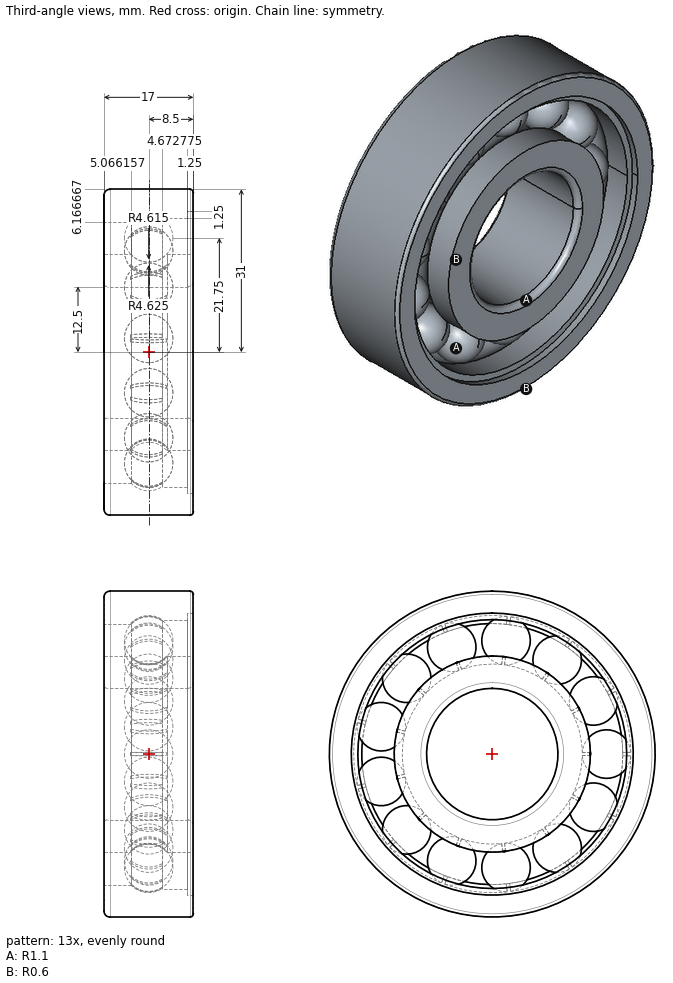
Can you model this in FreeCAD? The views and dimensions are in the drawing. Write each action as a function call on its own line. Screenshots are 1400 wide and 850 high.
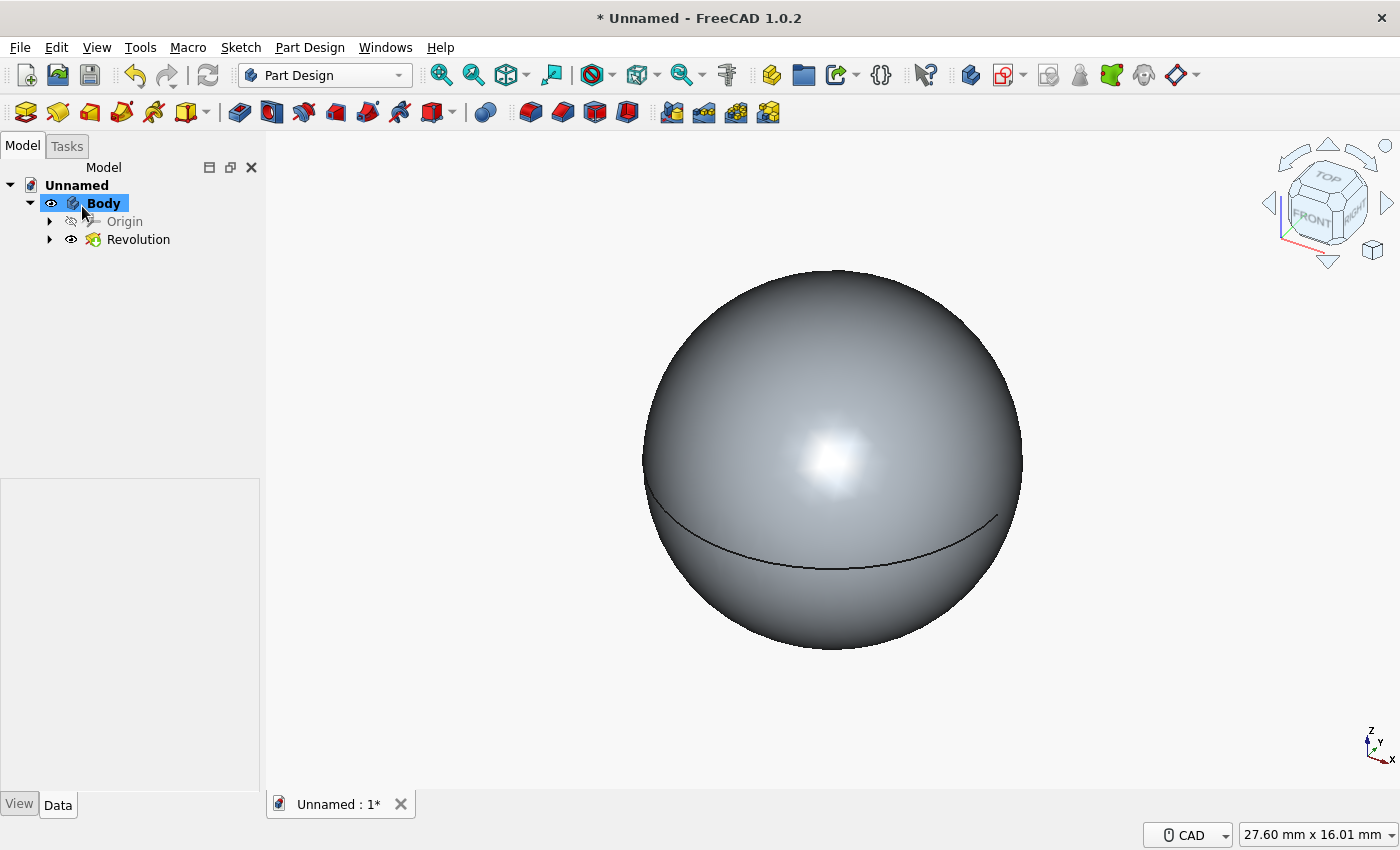
click(1004, 76)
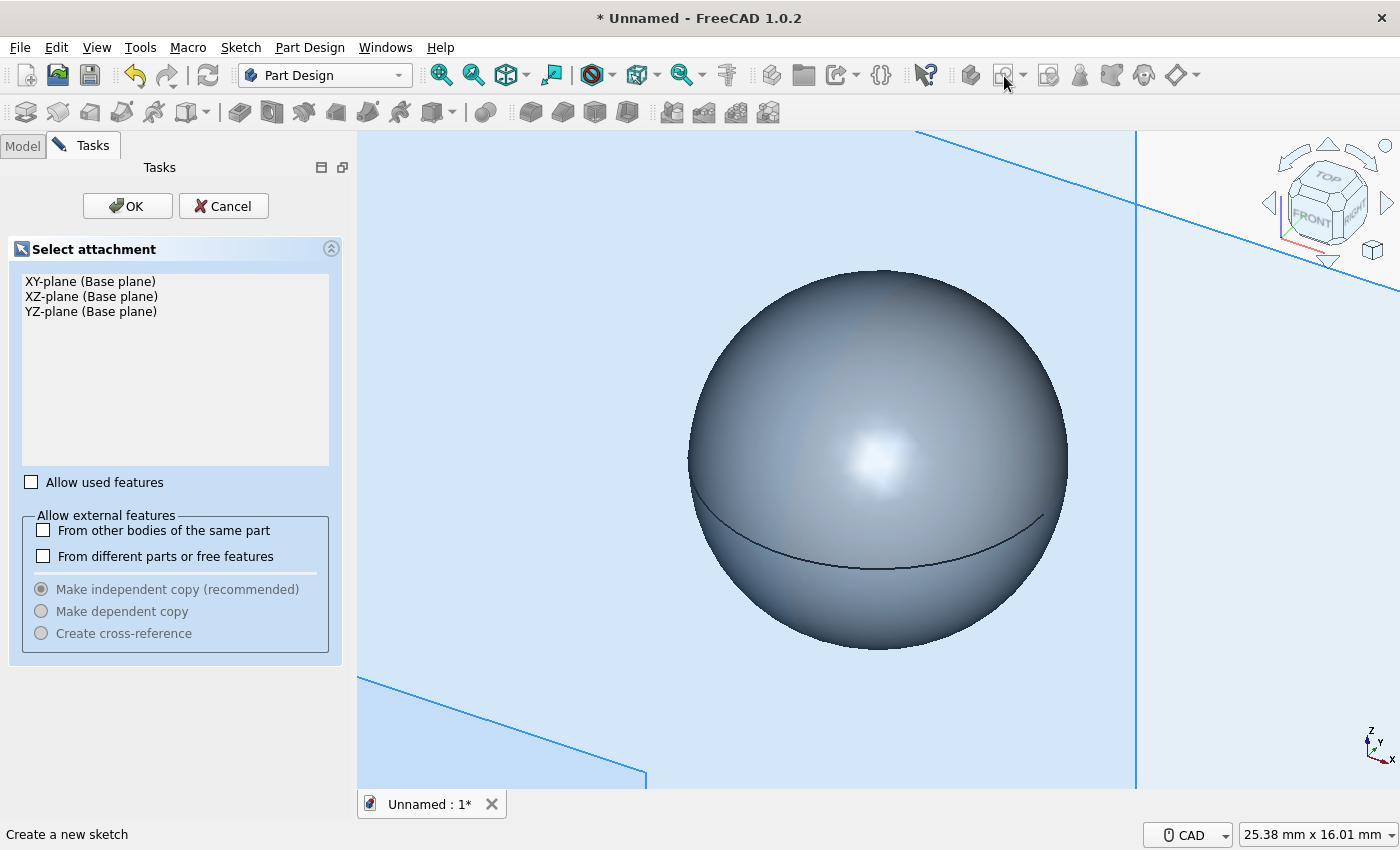
click(82, 282)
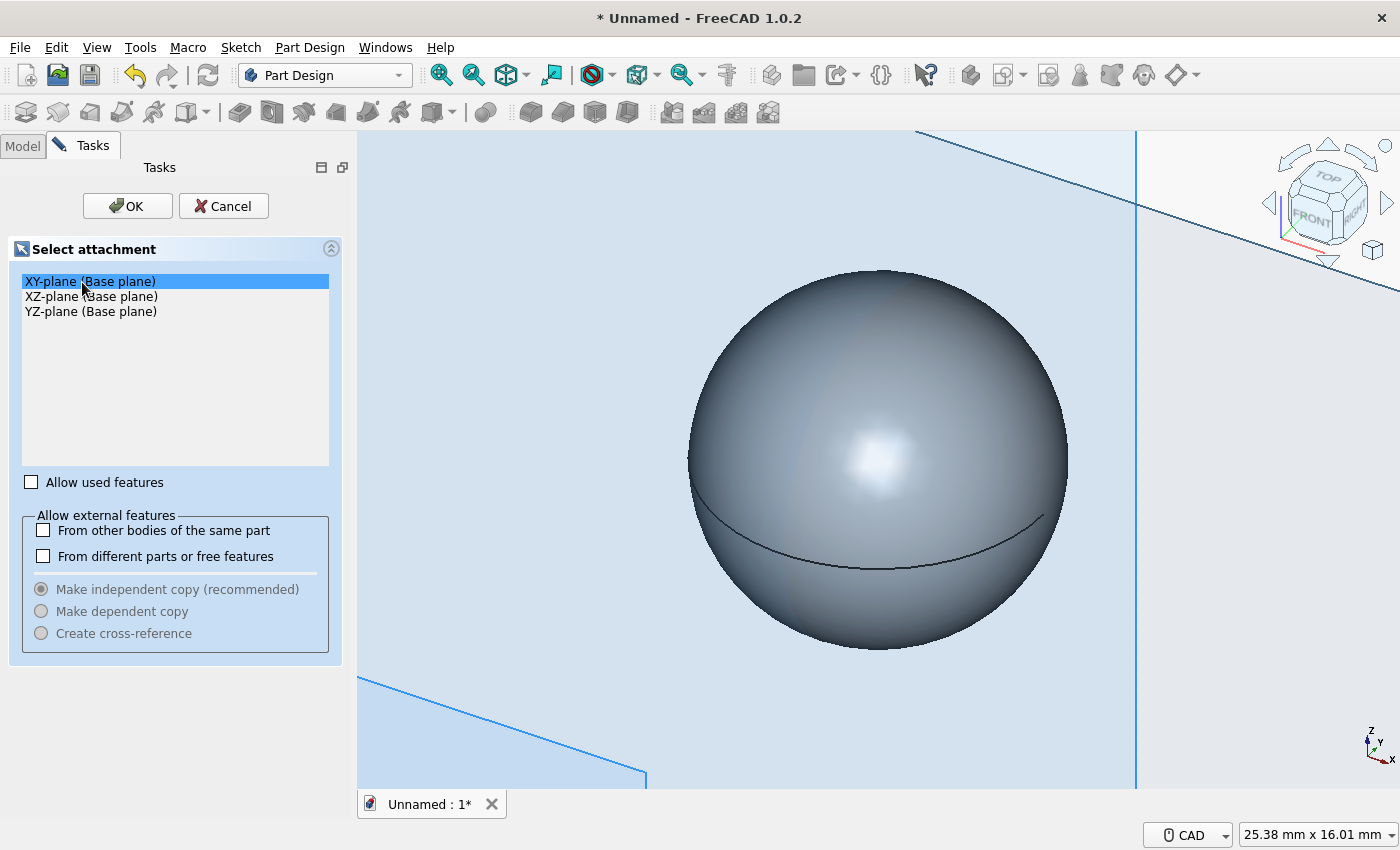
click(128, 206)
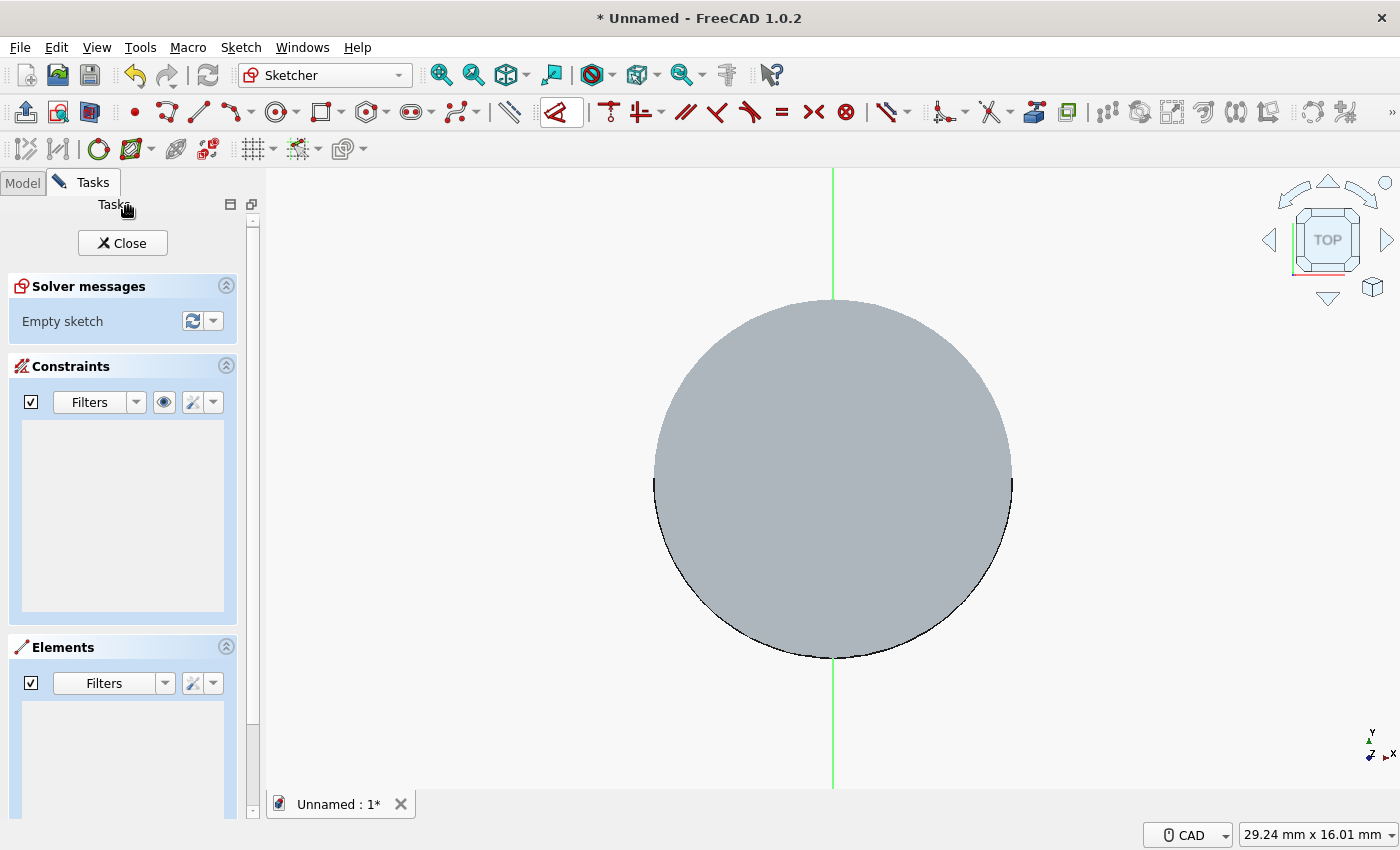
click(90, 112)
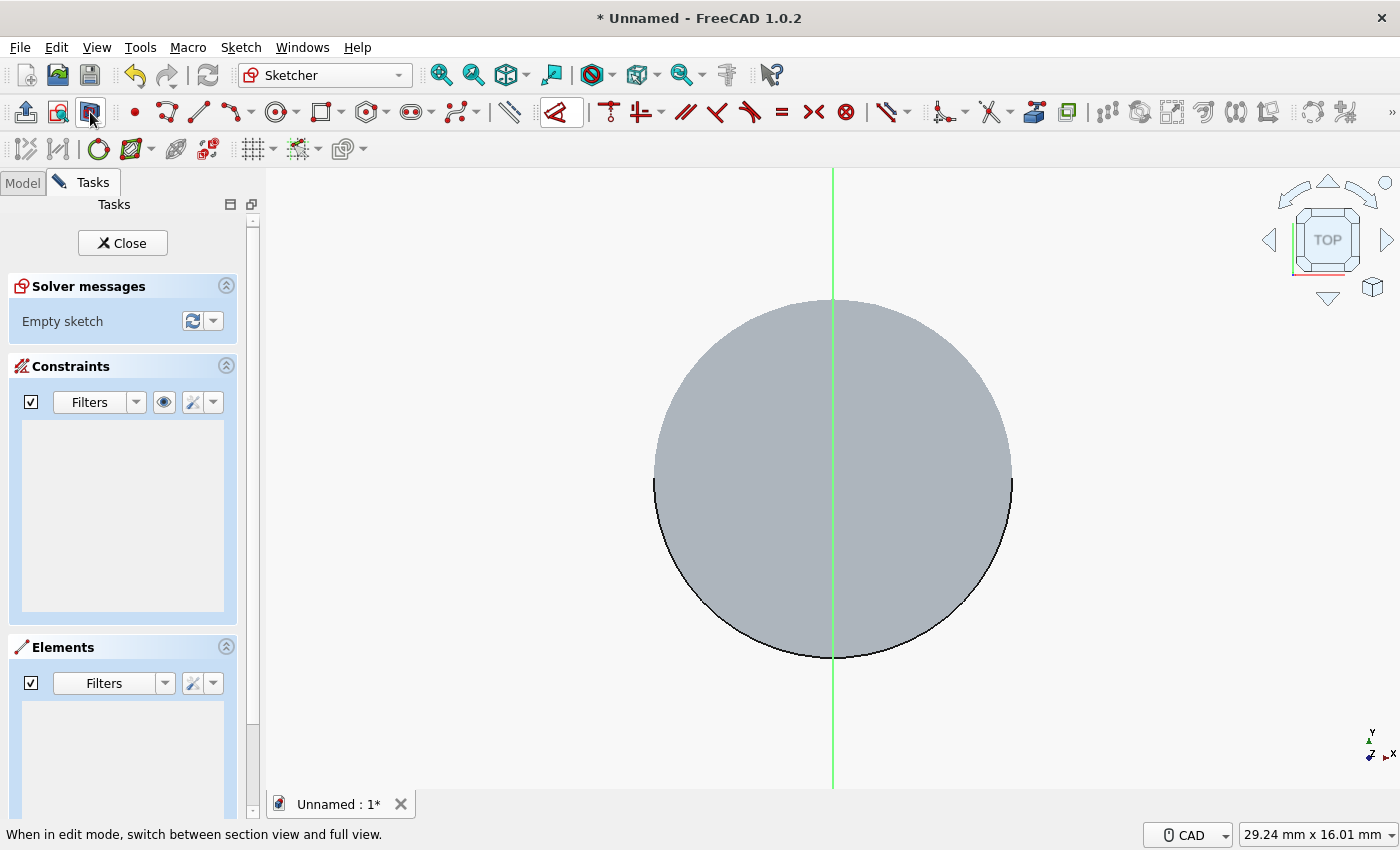
scroll(709, 196, down, 4)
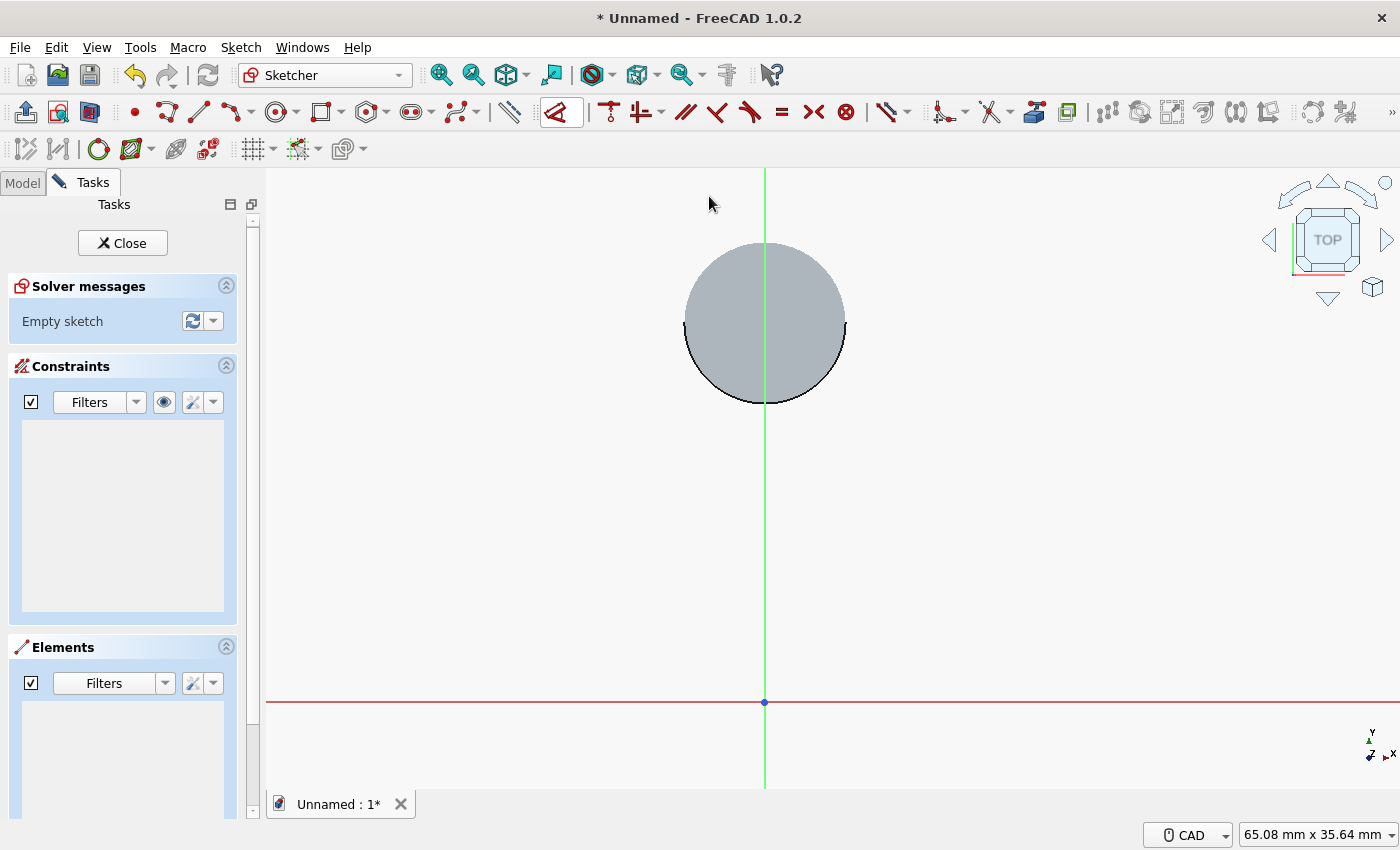
click(168, 112)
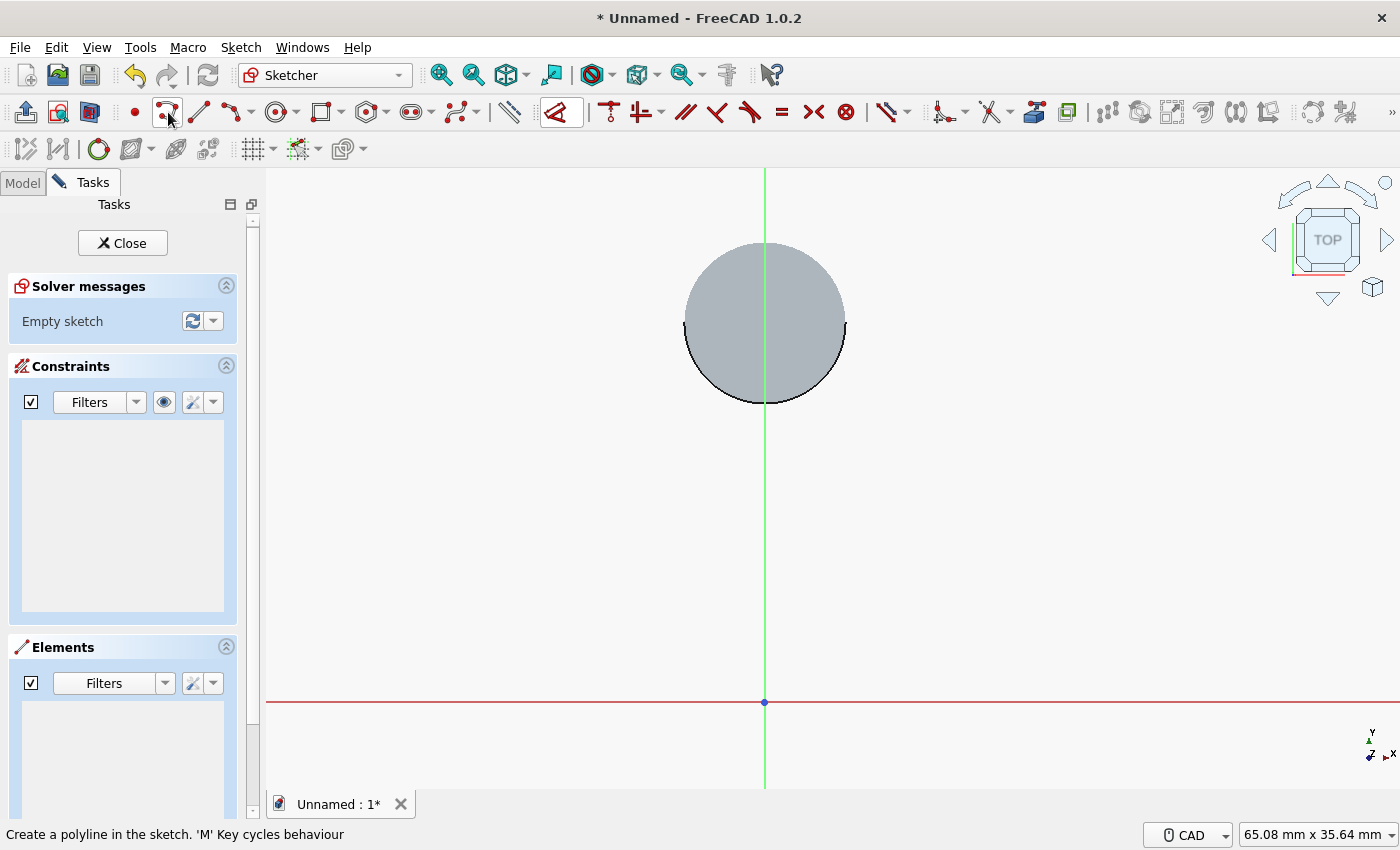
click(705, 377)
click(617, 377)
click(617, 484)
click(913, 484)
click(913, 377)
click(825, 377)
right_click(825, 377)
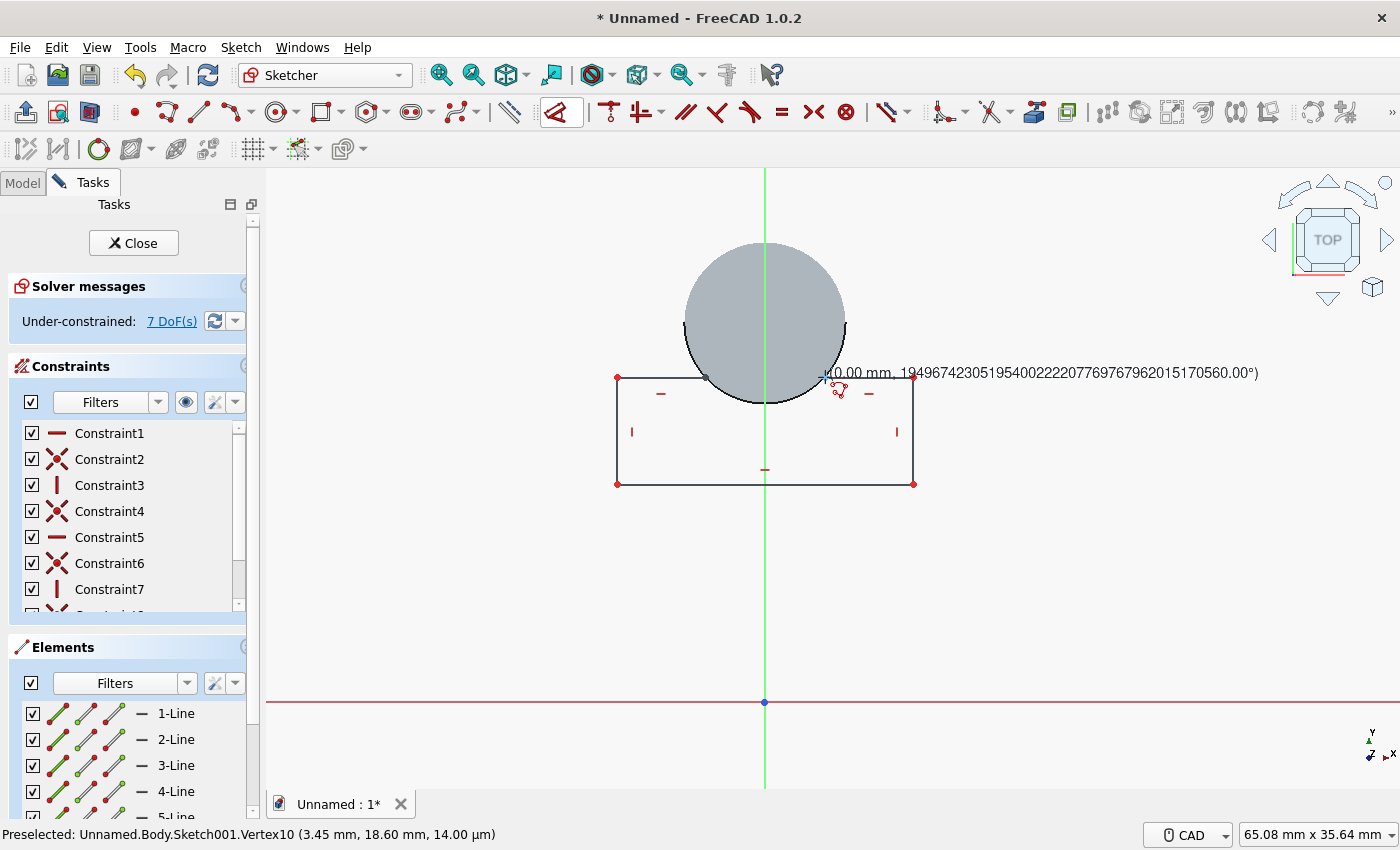
key(g)
key(3)
key(a)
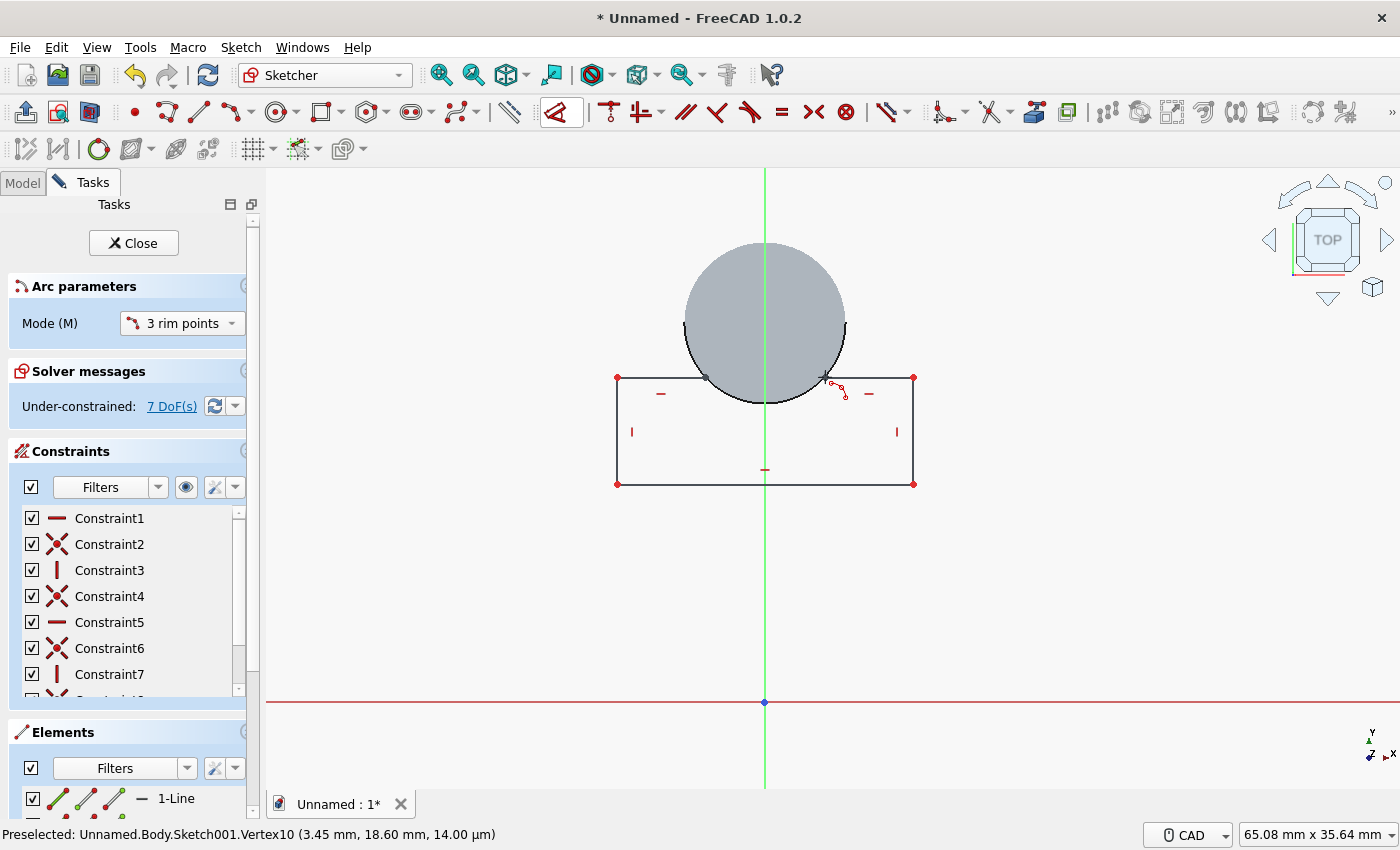
click(825, 378)
click(705, 378)
click(738, 399)
key(Escape)